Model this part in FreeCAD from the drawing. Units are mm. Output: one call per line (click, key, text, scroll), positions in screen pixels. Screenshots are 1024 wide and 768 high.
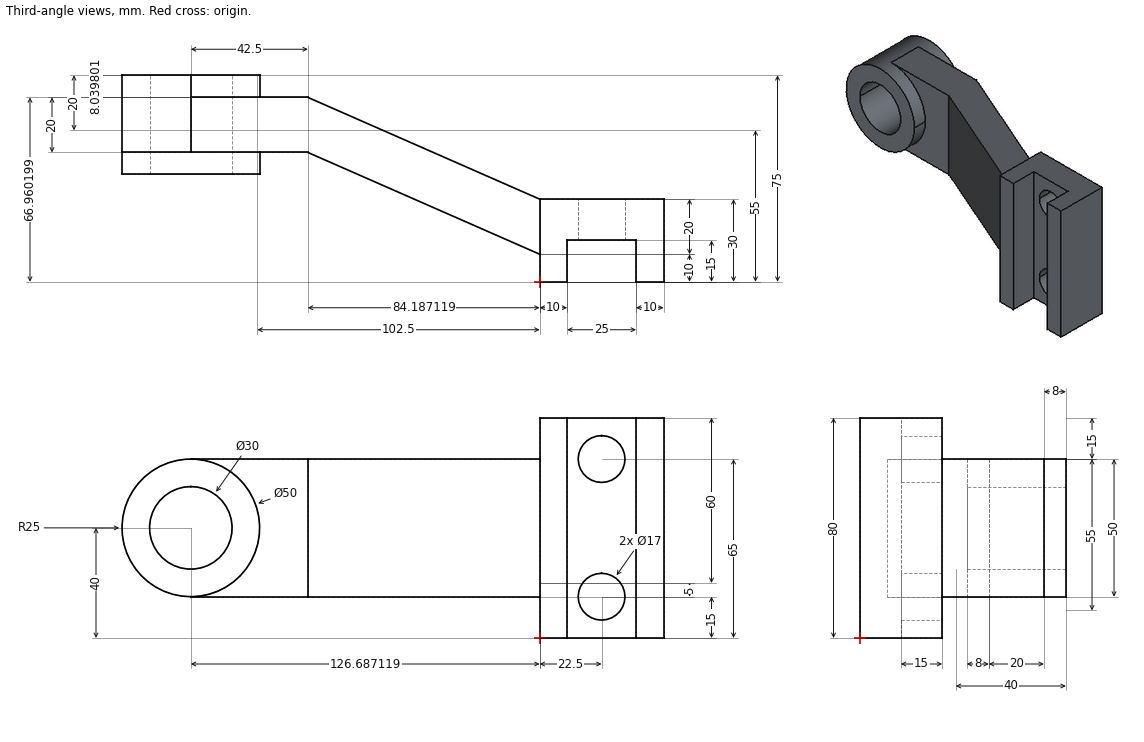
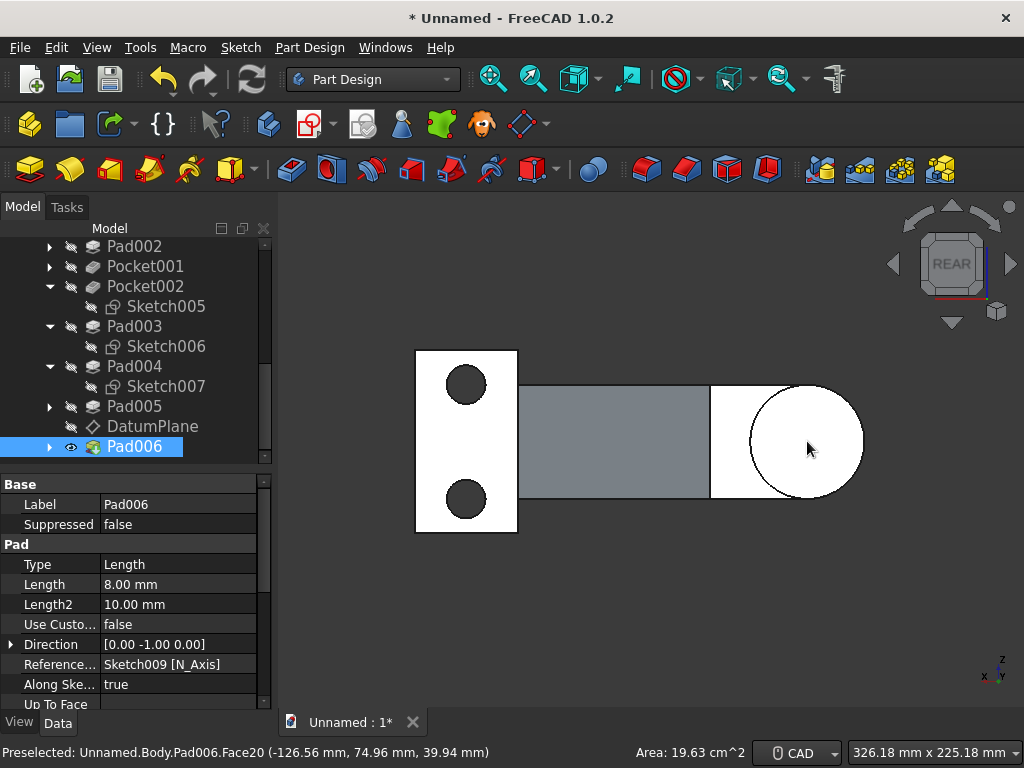
click(310, 124)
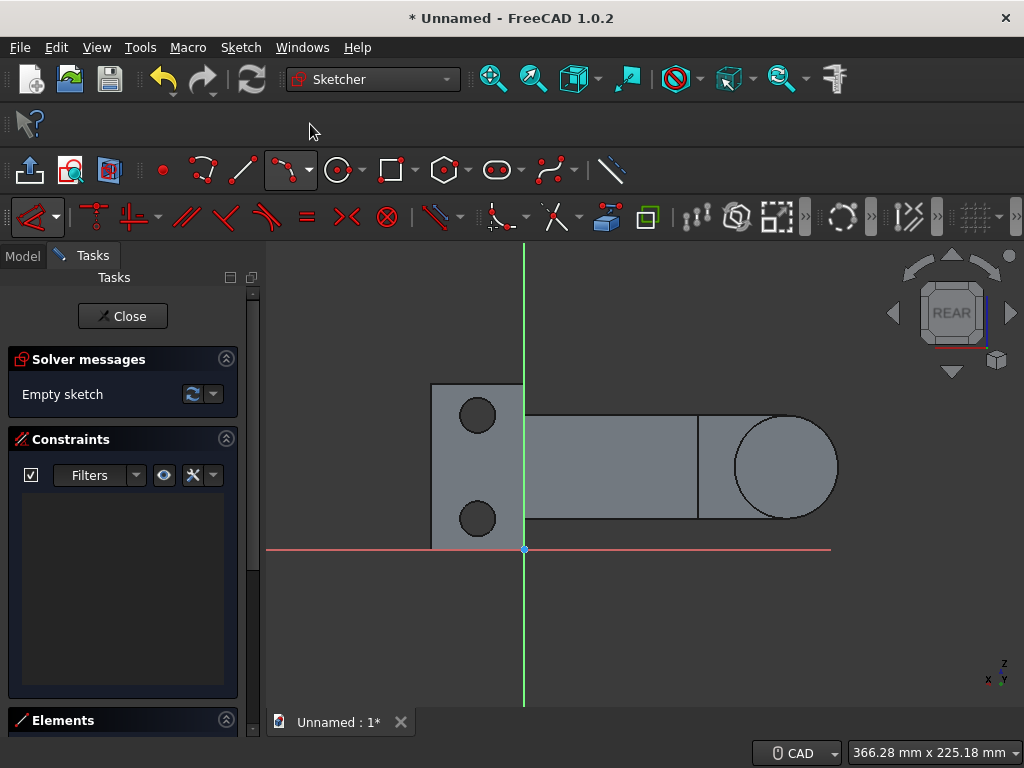
scroll(840, 465, up, 8)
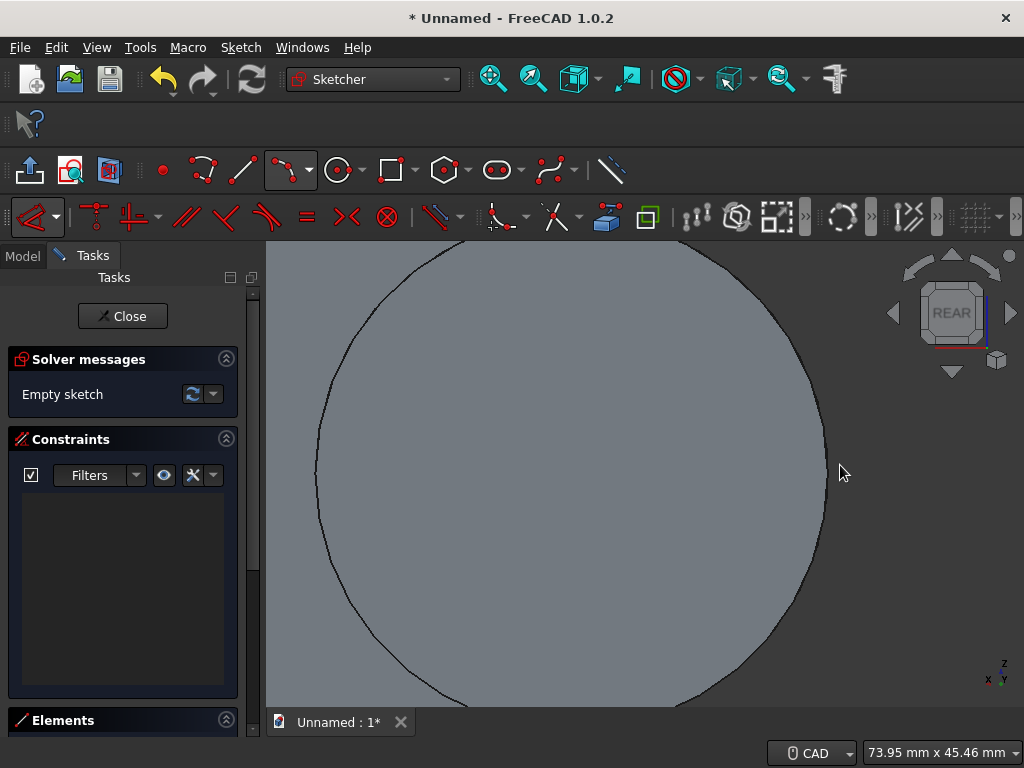
key(g)
key(c)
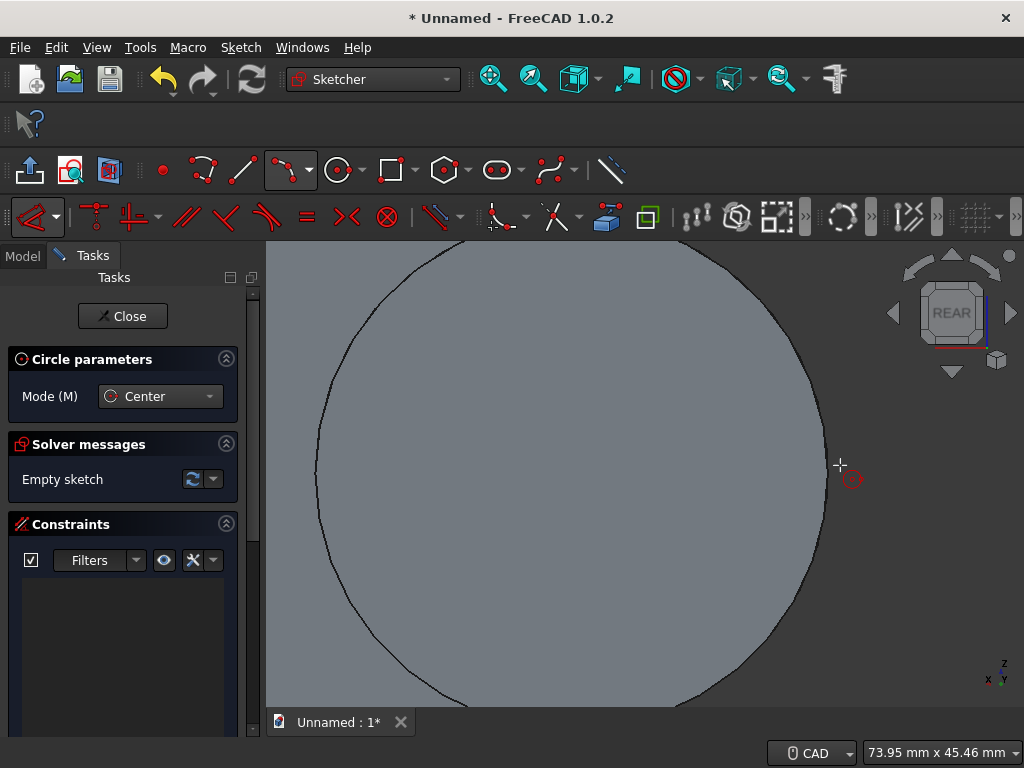
click(572, 473)
move(680, 365)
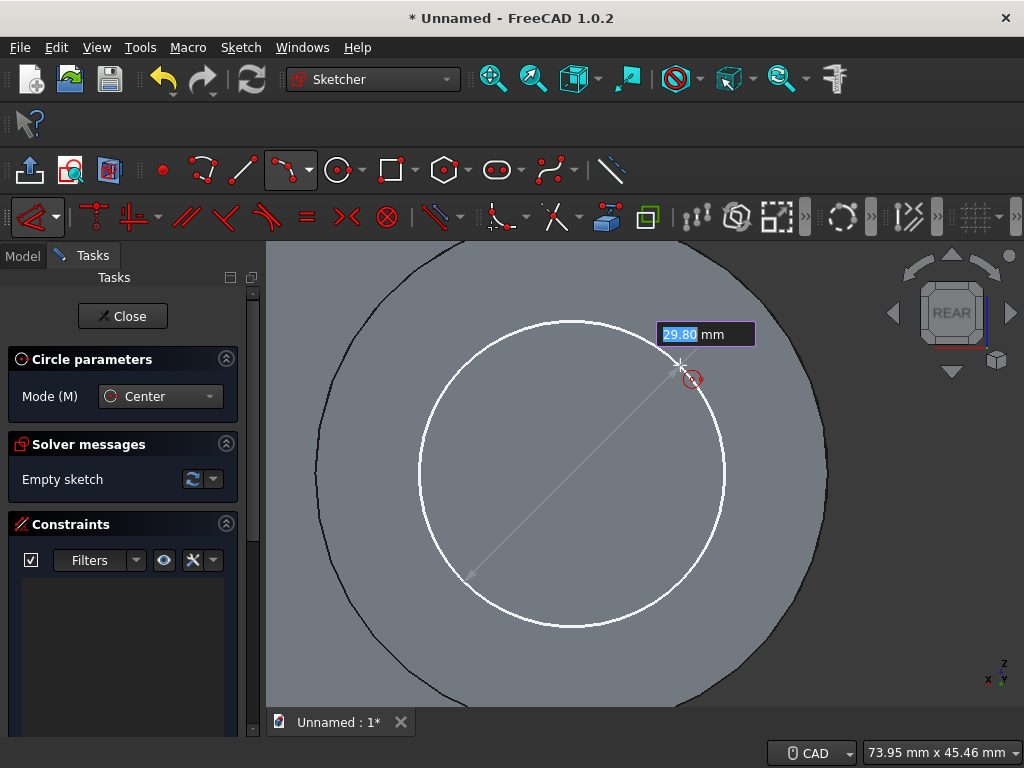
text(30)
key(Return)
key(Escape)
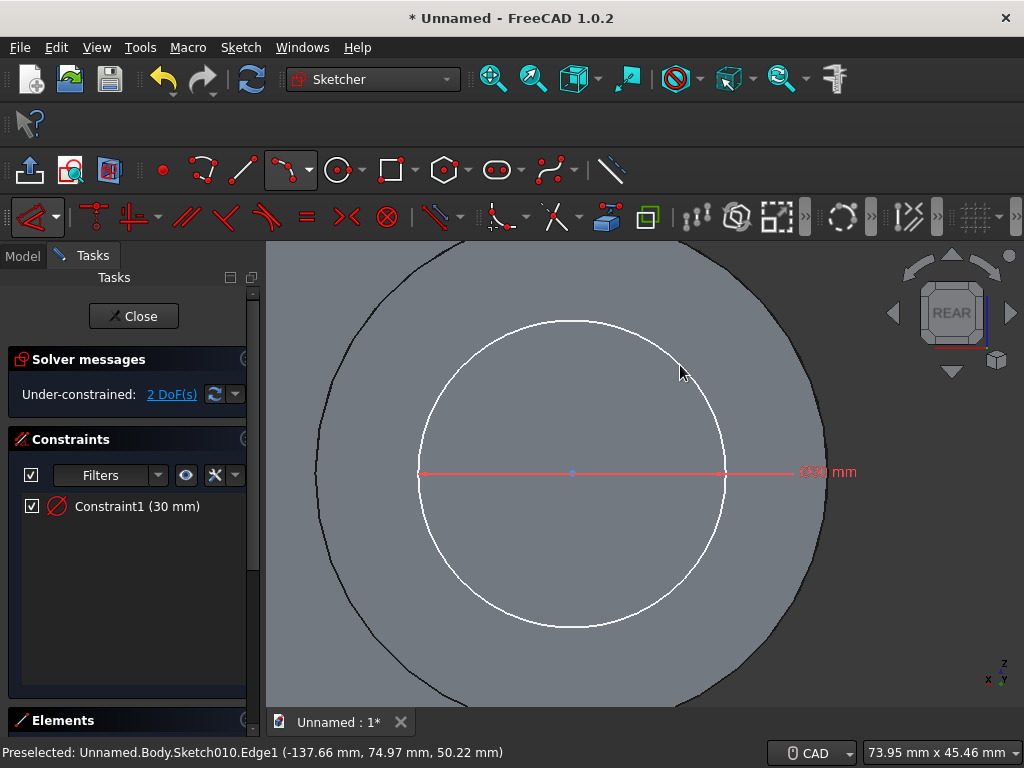
click(572, 474)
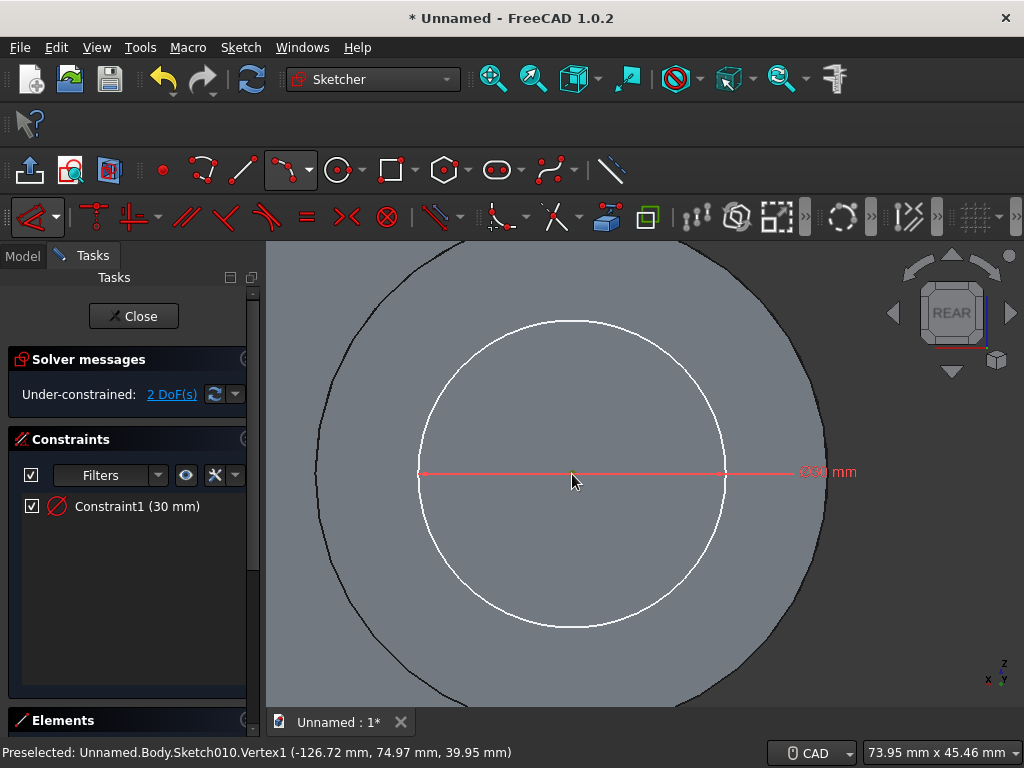
key(i)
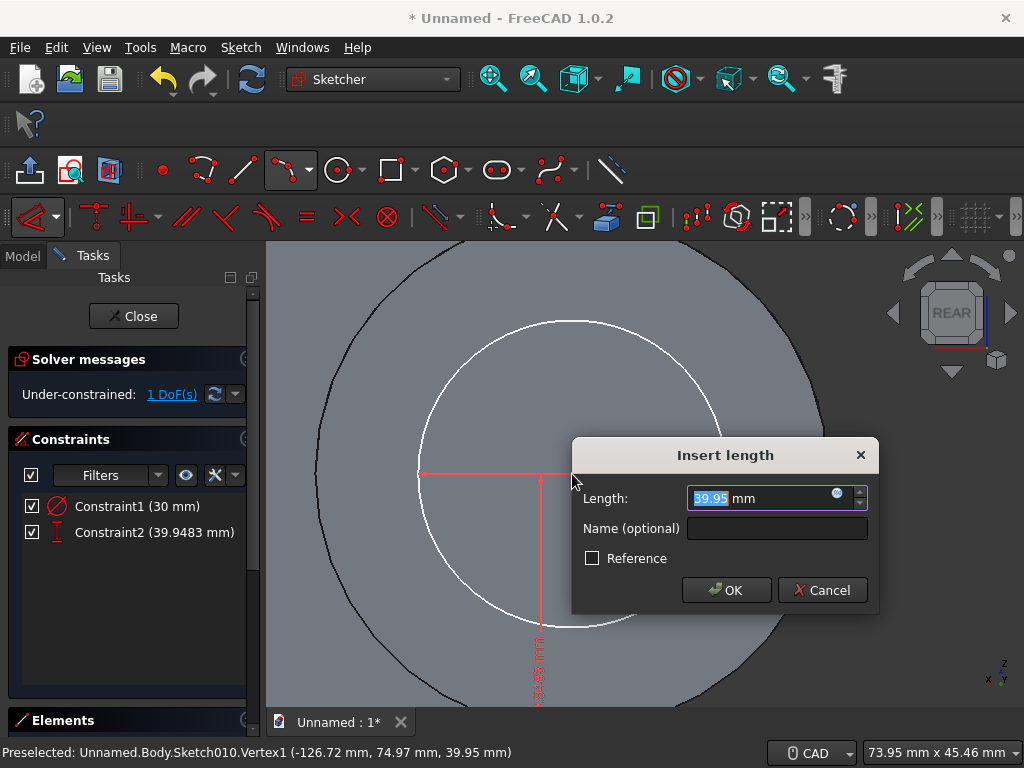
text(40)
key(Return)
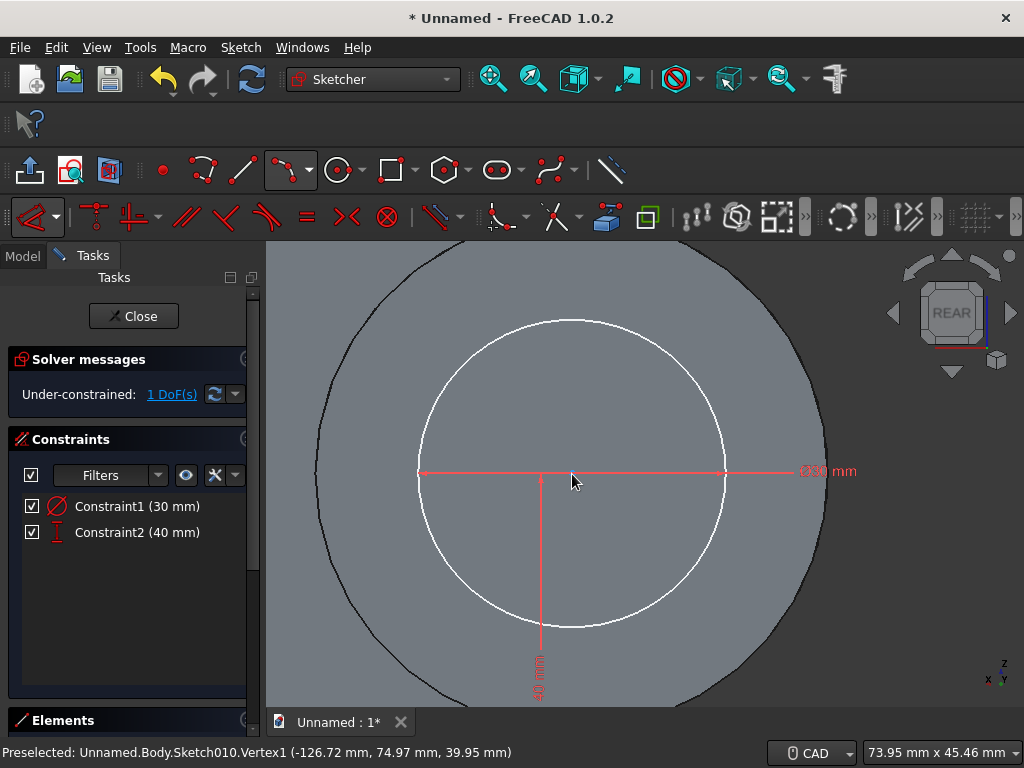
click(572, 473)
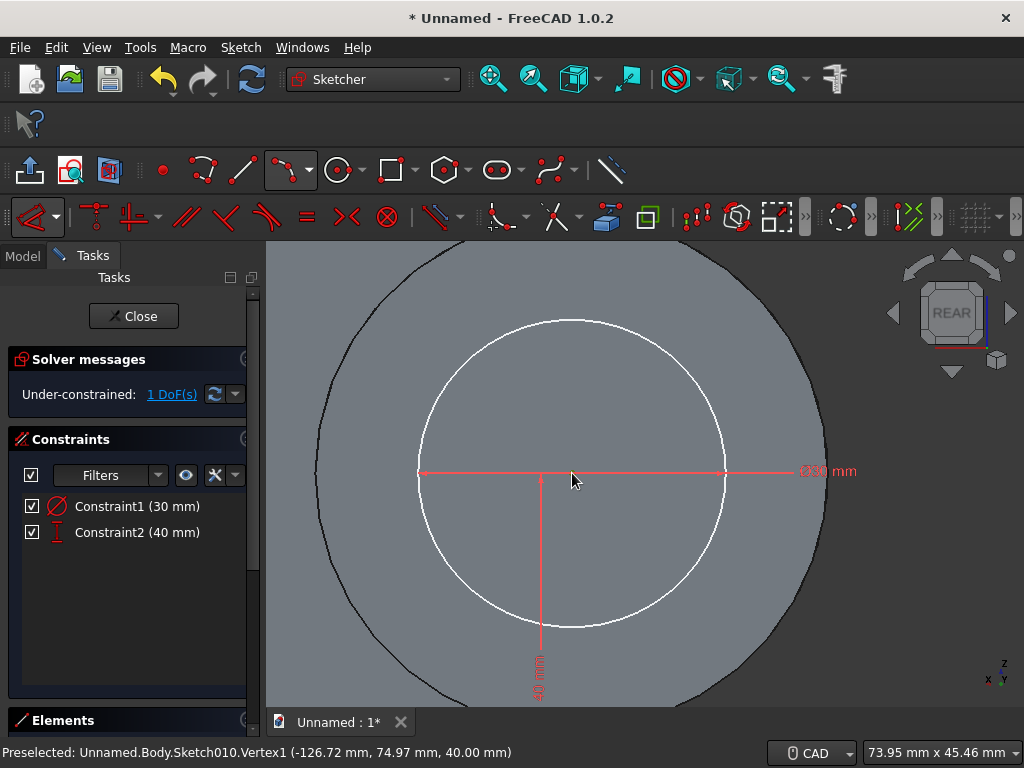
key(l)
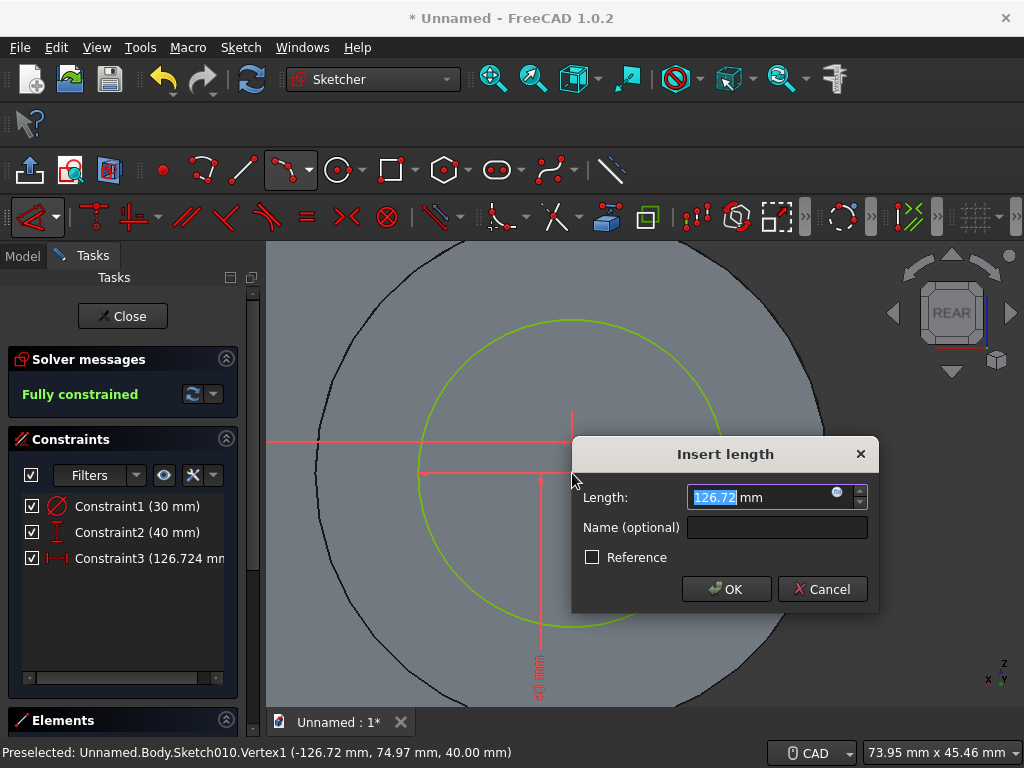
text(126.687119)
key(Return)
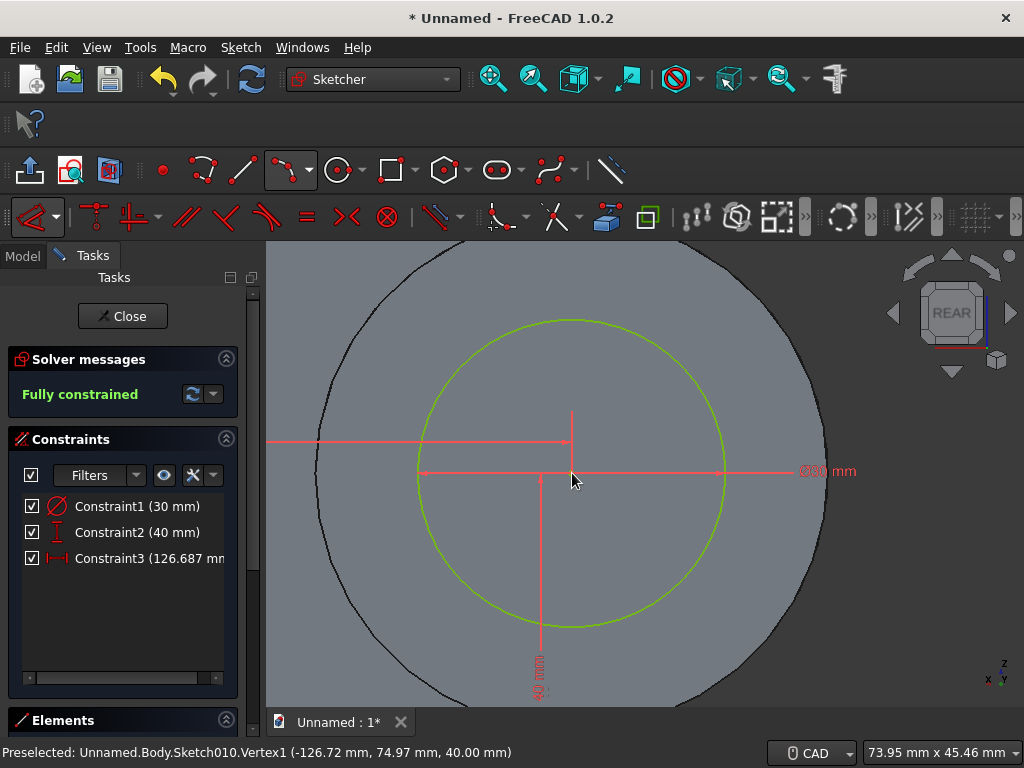
click(123, 316)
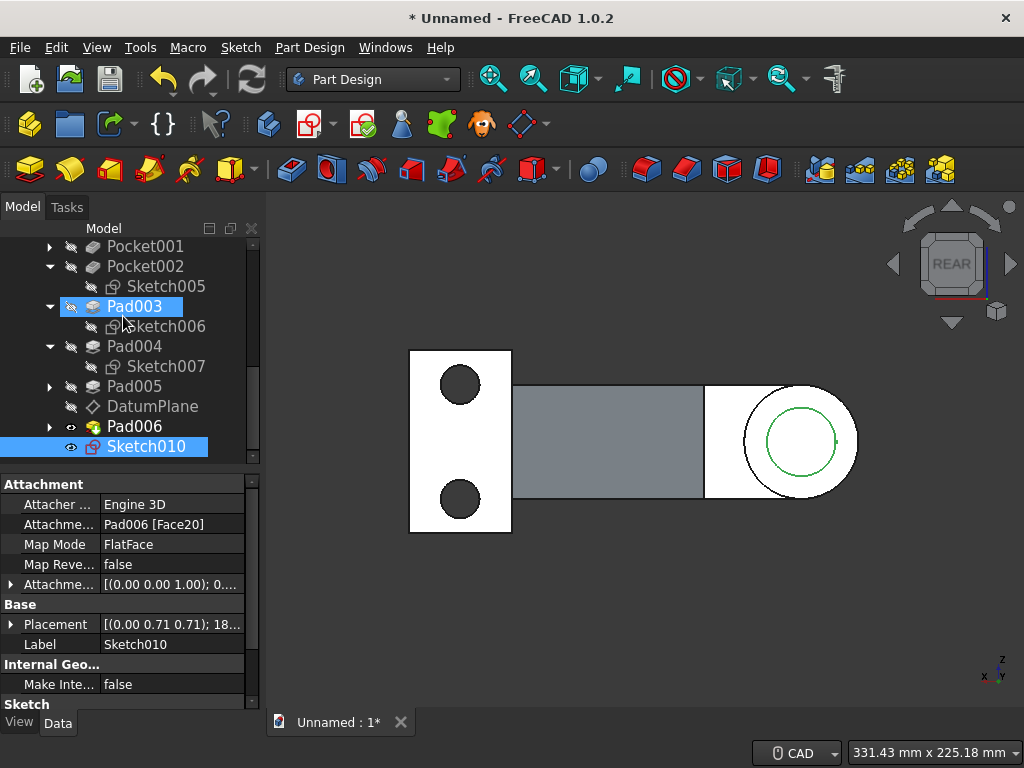
click(292, 170)